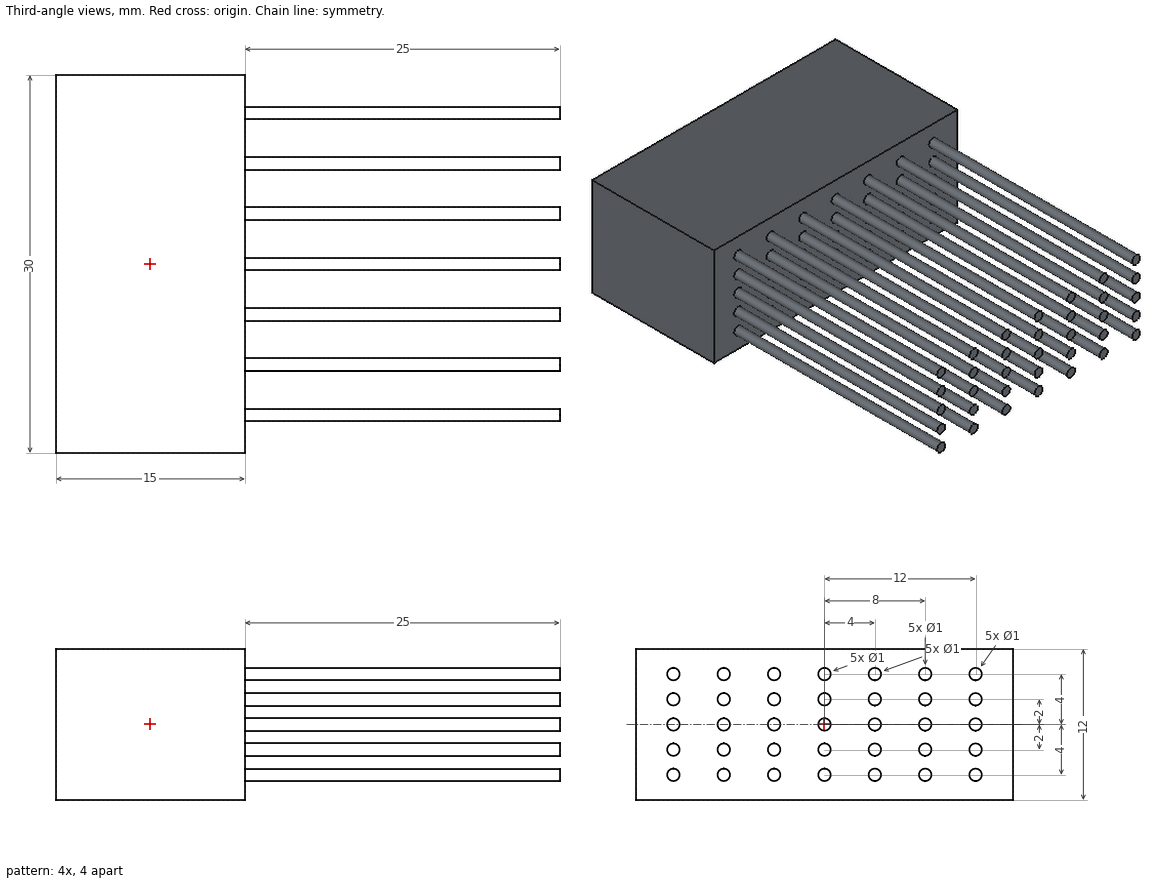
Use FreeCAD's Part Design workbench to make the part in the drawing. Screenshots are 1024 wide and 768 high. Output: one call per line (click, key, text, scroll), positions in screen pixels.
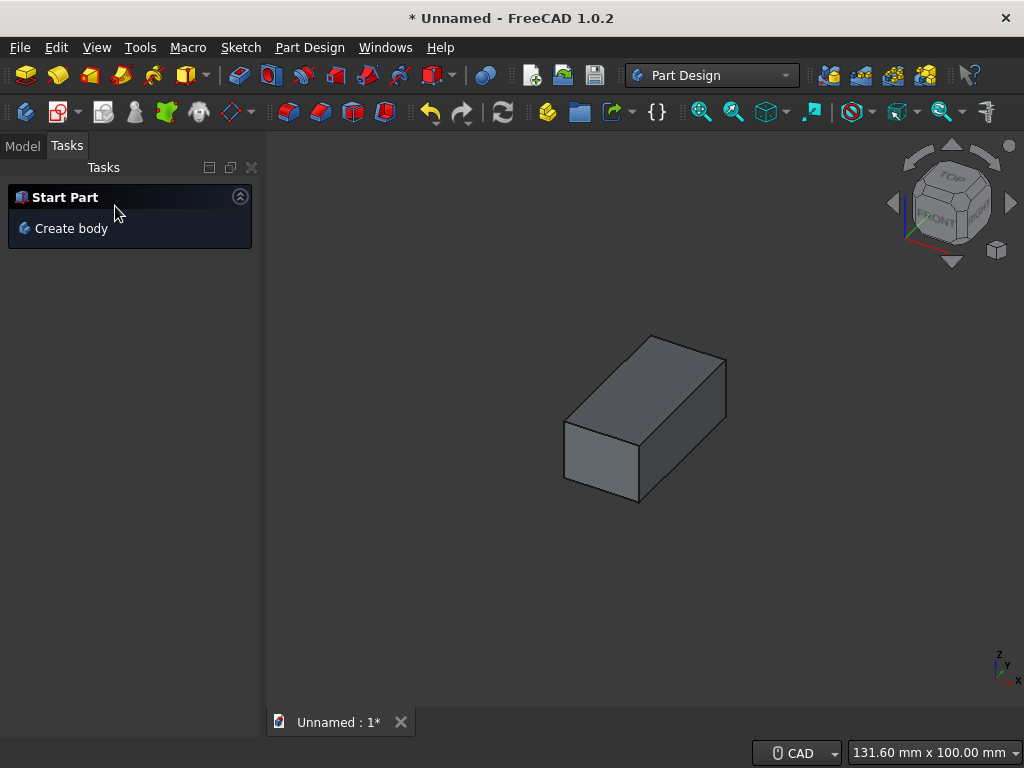
key(v)
key(f)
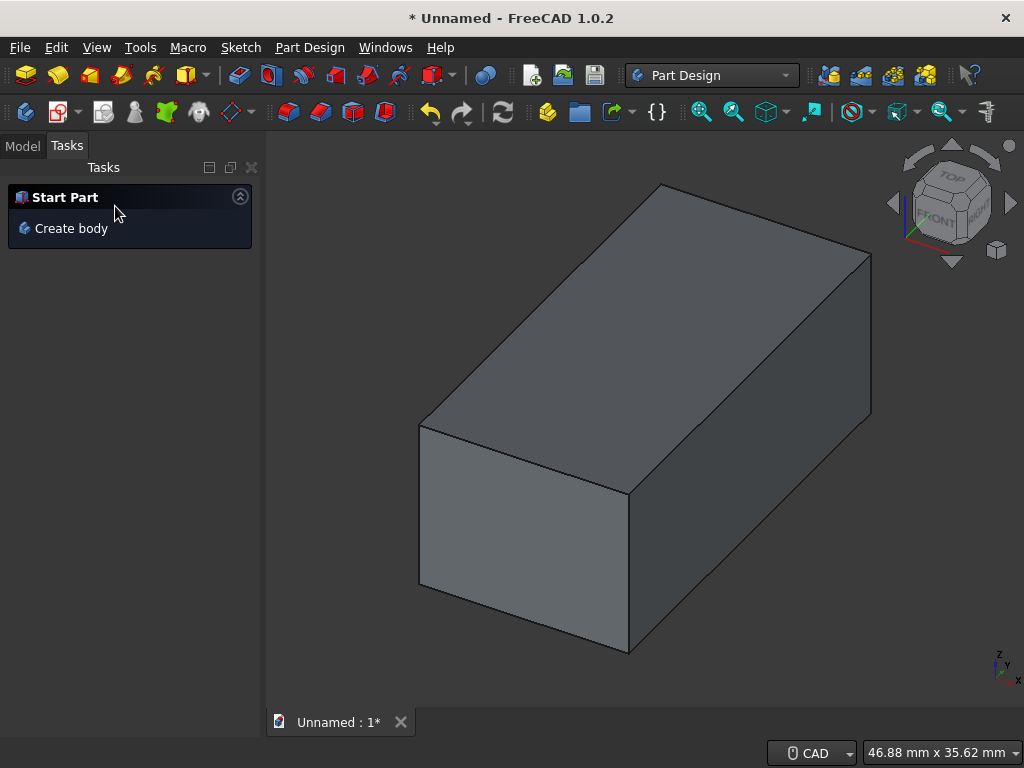
click(819, 384)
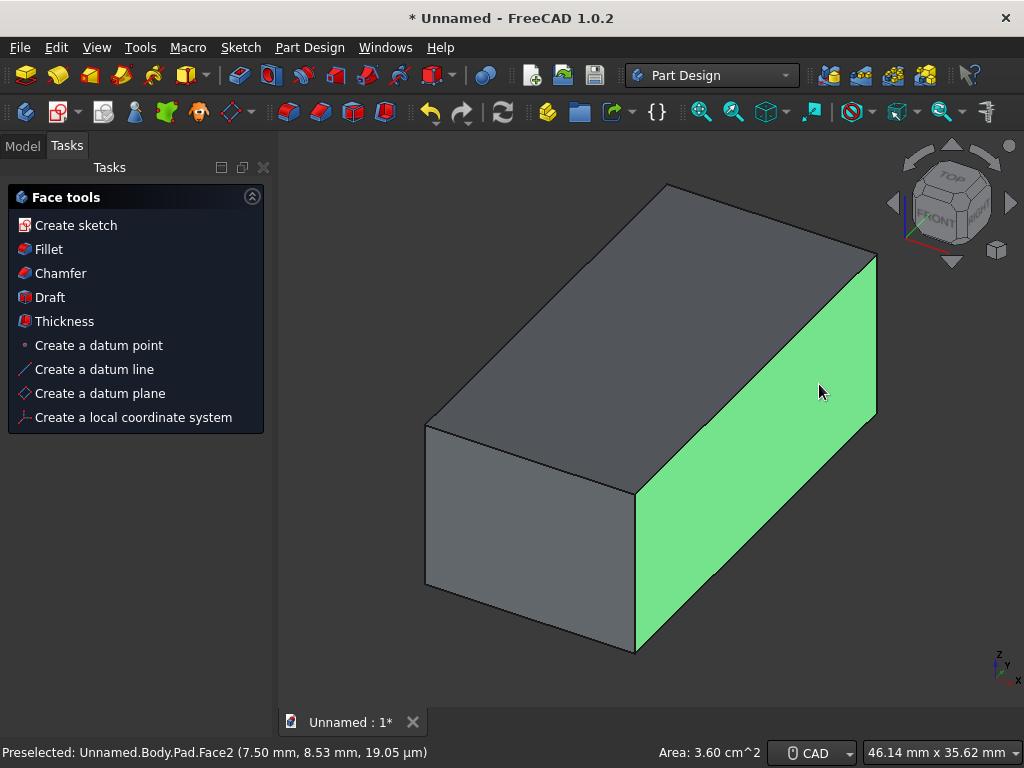
click(58, 112)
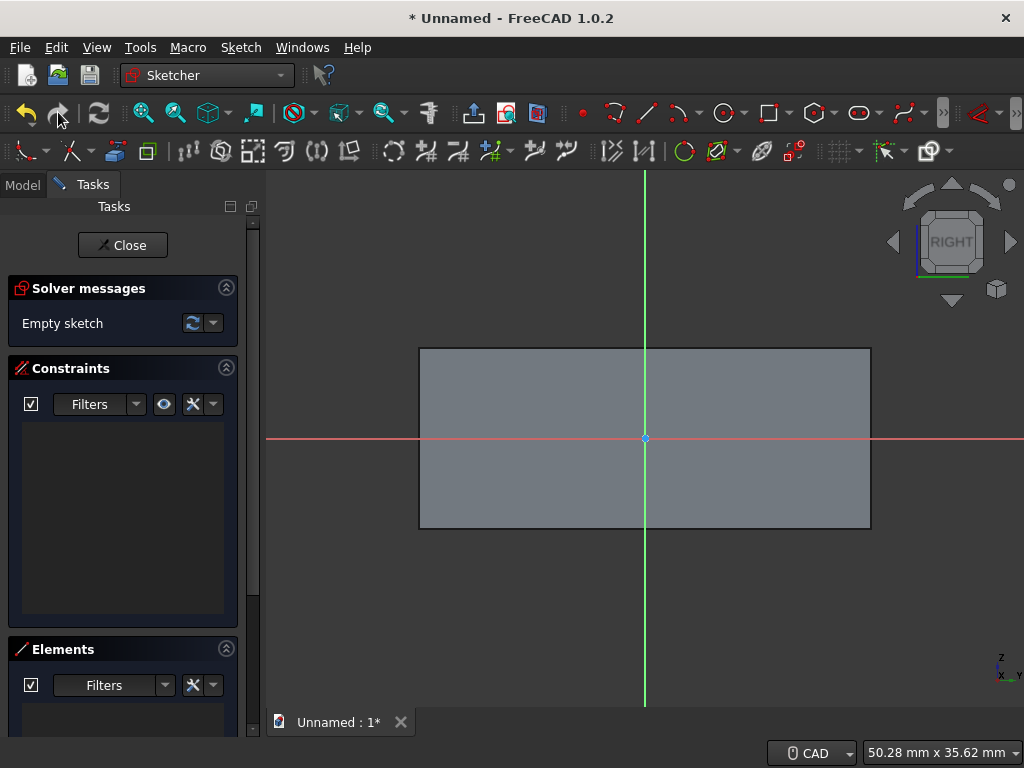
scroll(685, 439, up, 5)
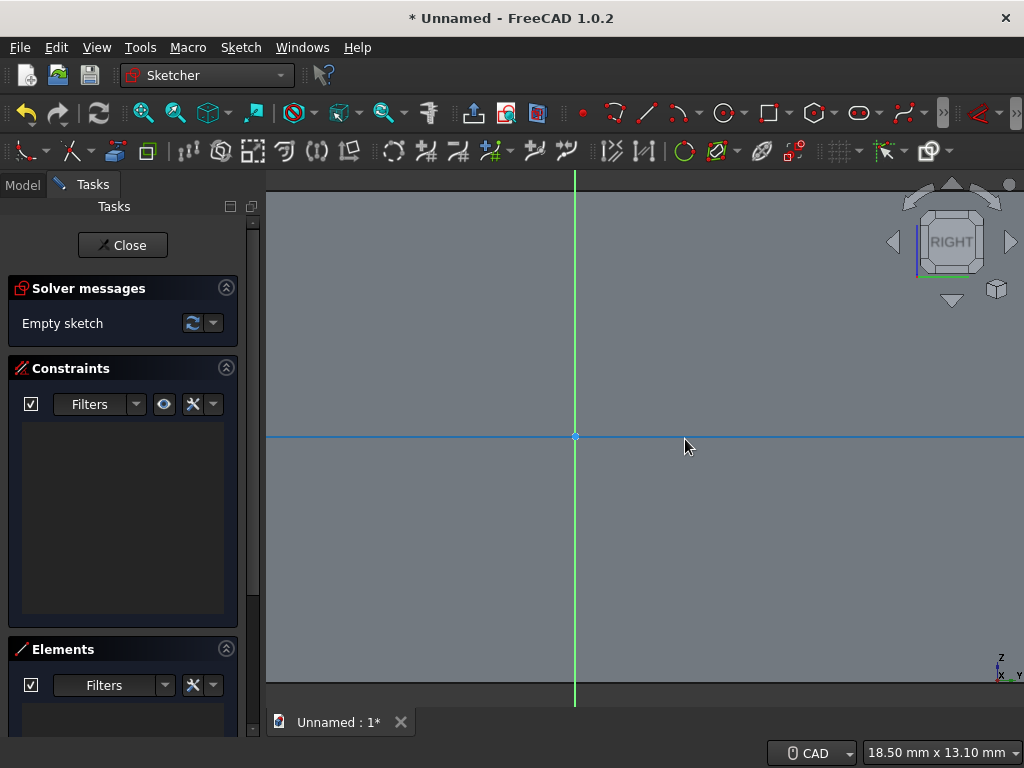
key(g)
key(c)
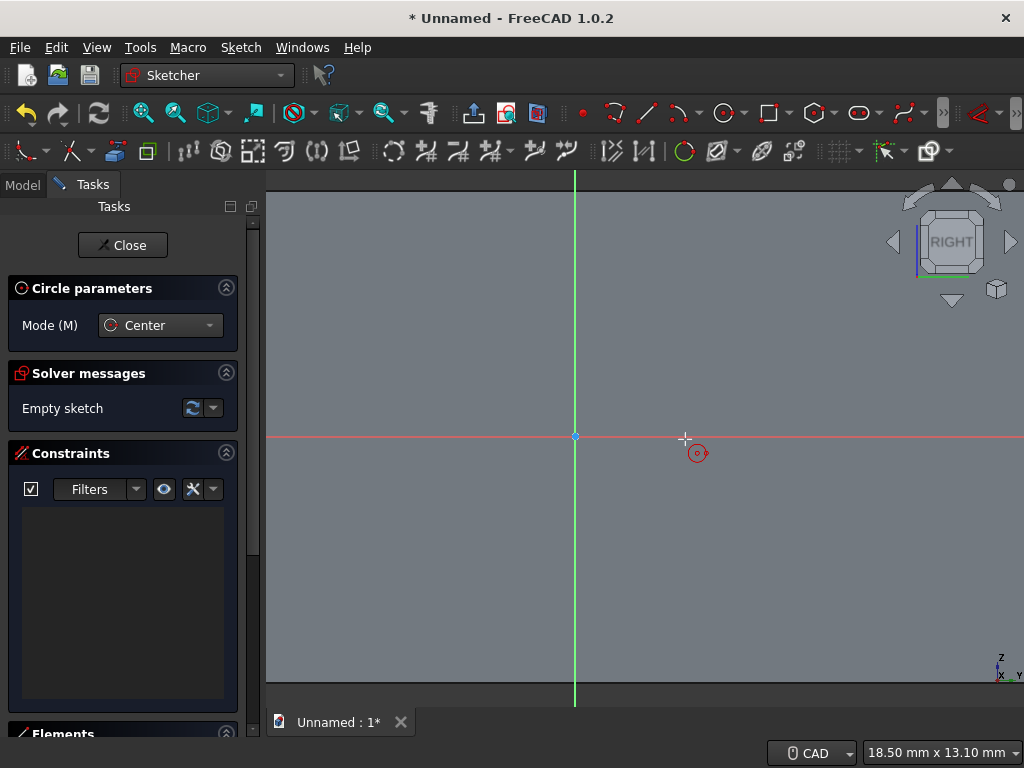
click(575, 273)
move(590, 258)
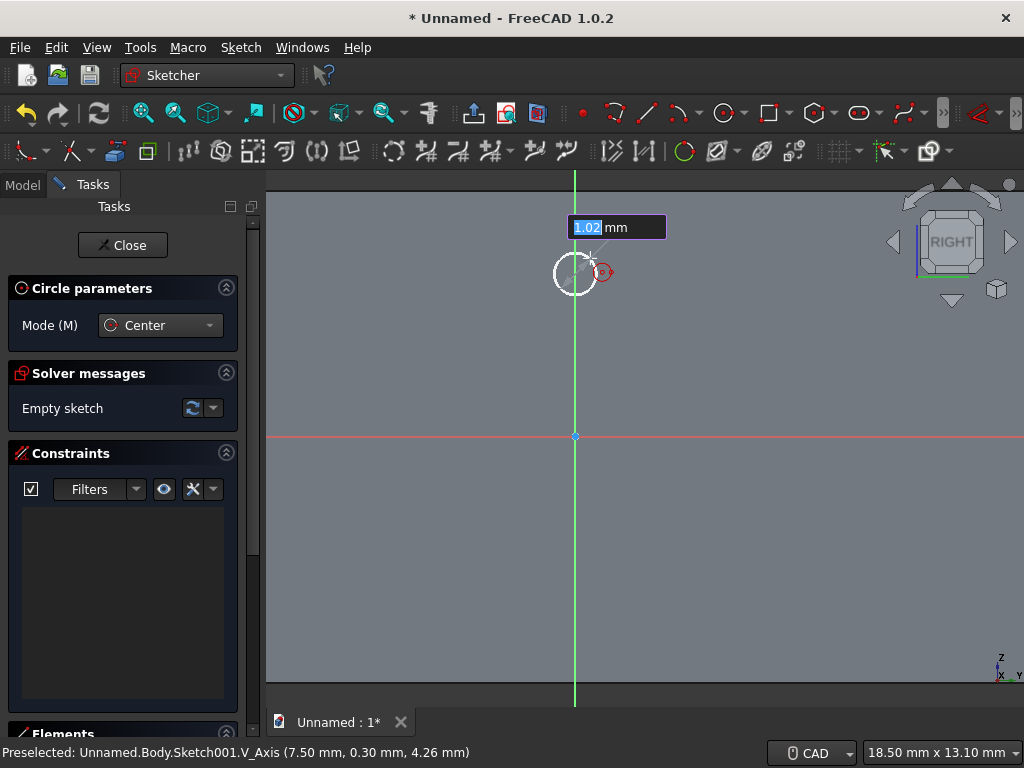
text(1)
key(Return)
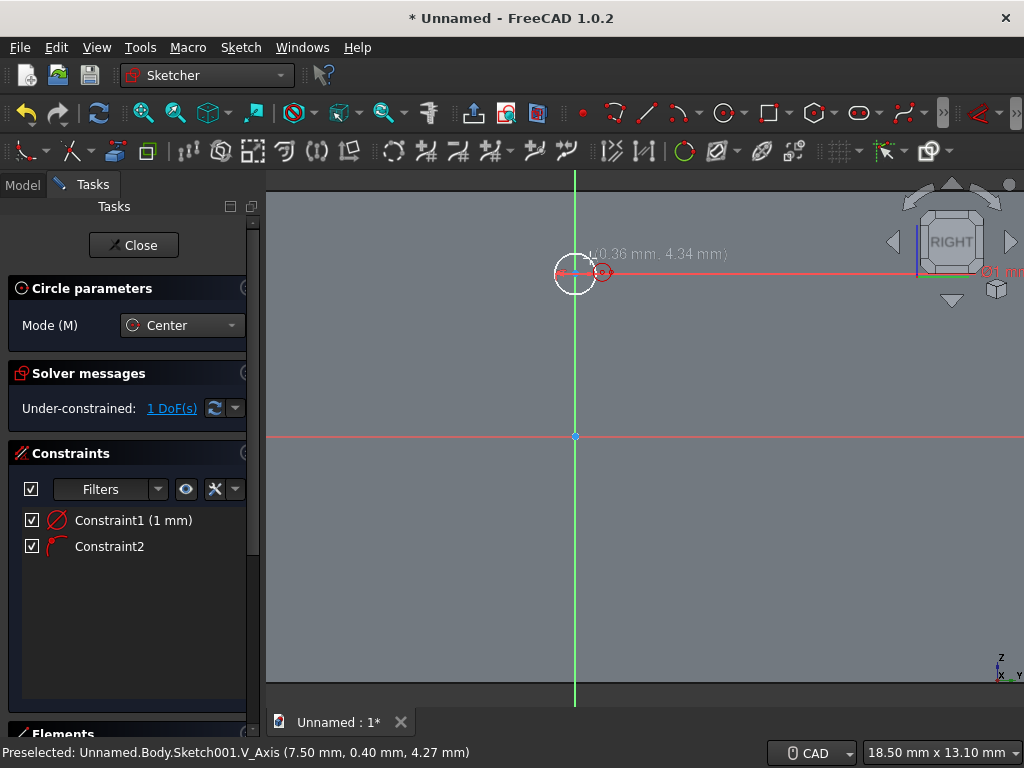
click(575, 355)
move(590, 340)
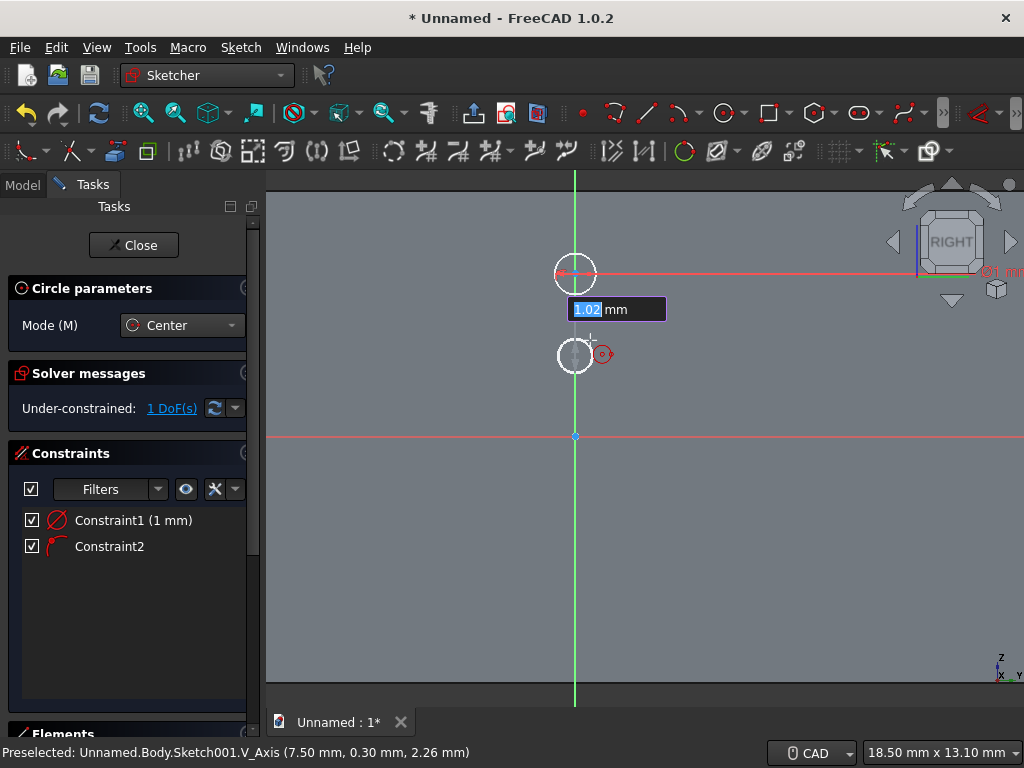
text(1)
key(Return)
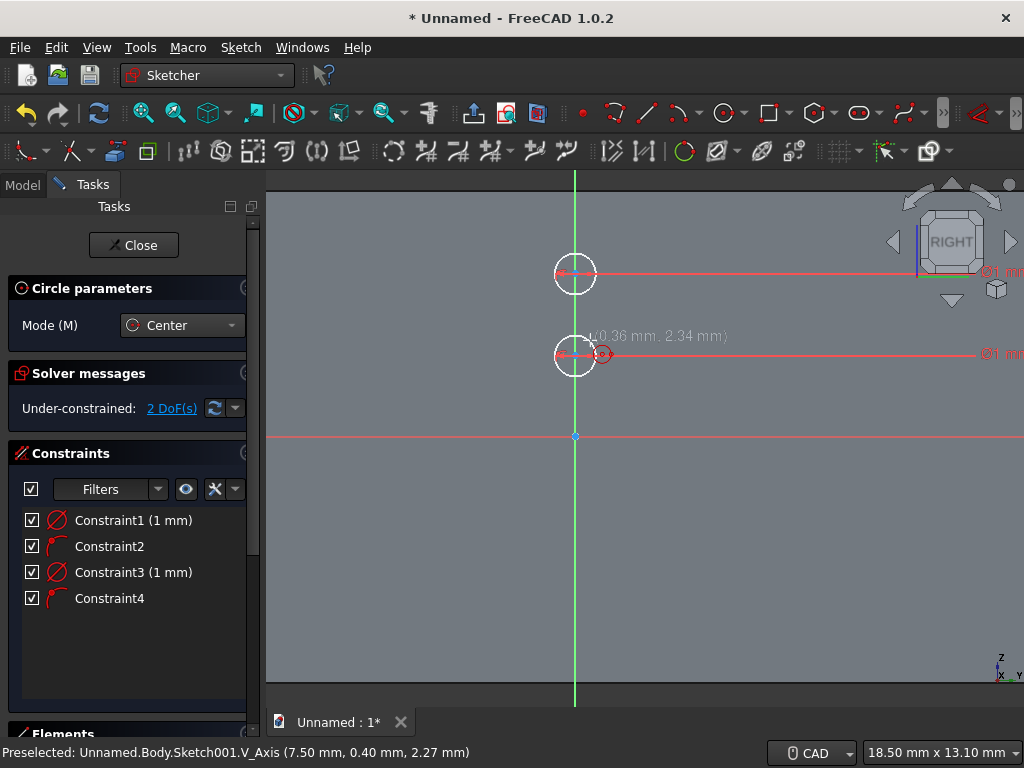
click(575, 437)
move(590, 422)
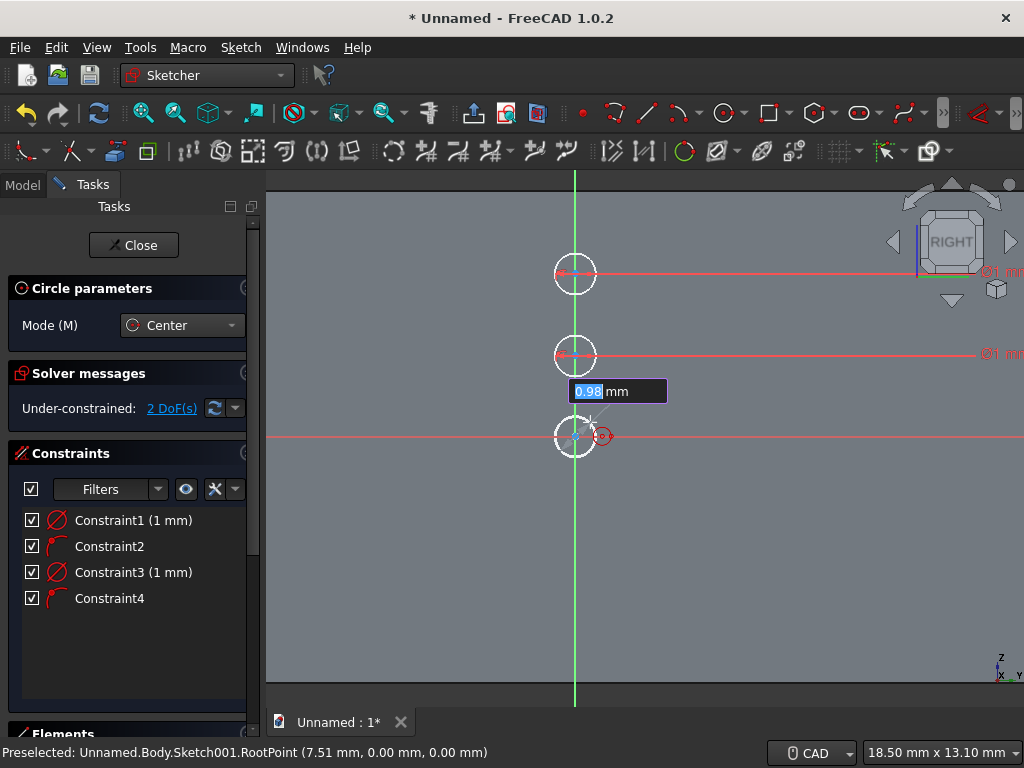
text(1)
key(Return)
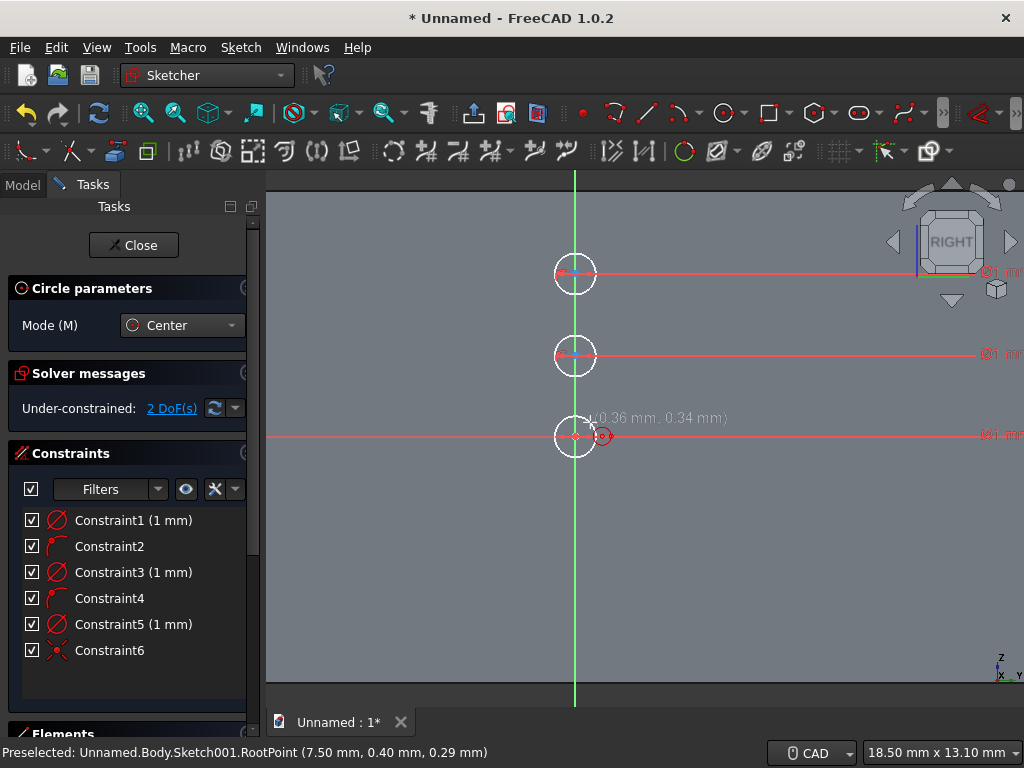
click(575, 519)
move(590, 504)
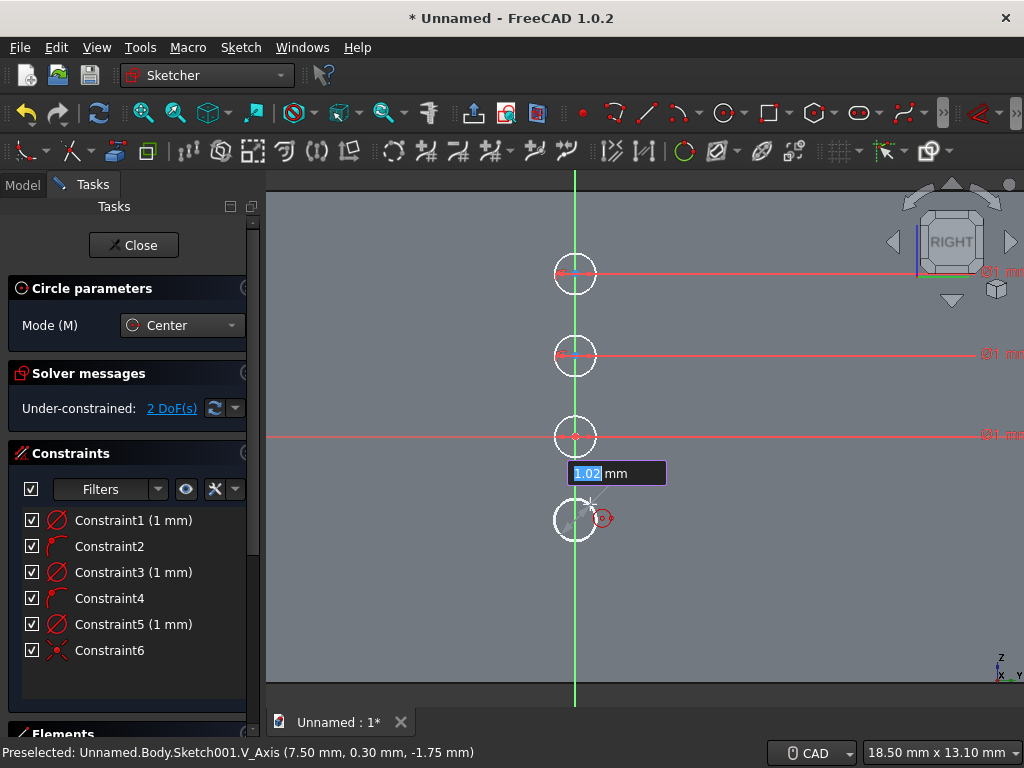
text(1)
key(Return)